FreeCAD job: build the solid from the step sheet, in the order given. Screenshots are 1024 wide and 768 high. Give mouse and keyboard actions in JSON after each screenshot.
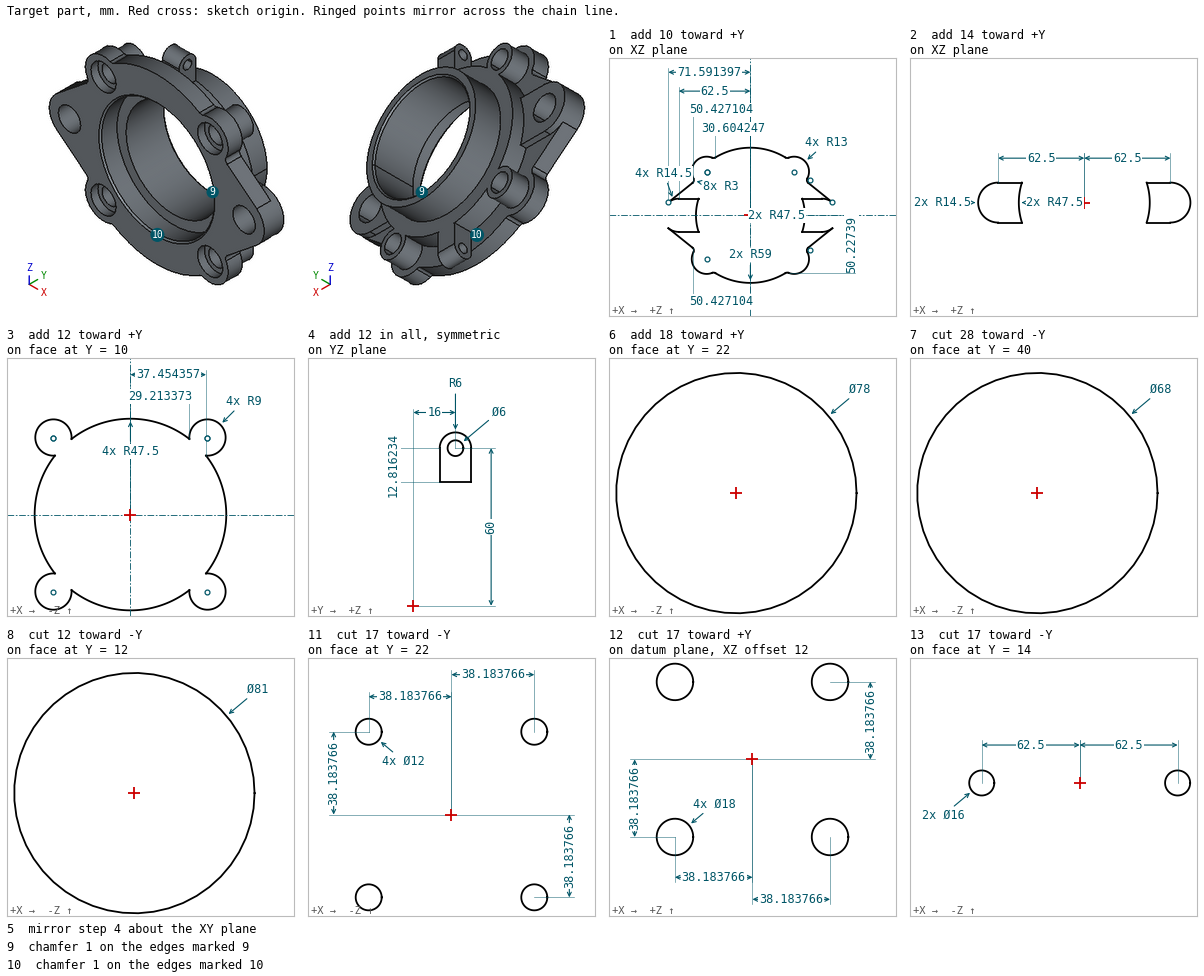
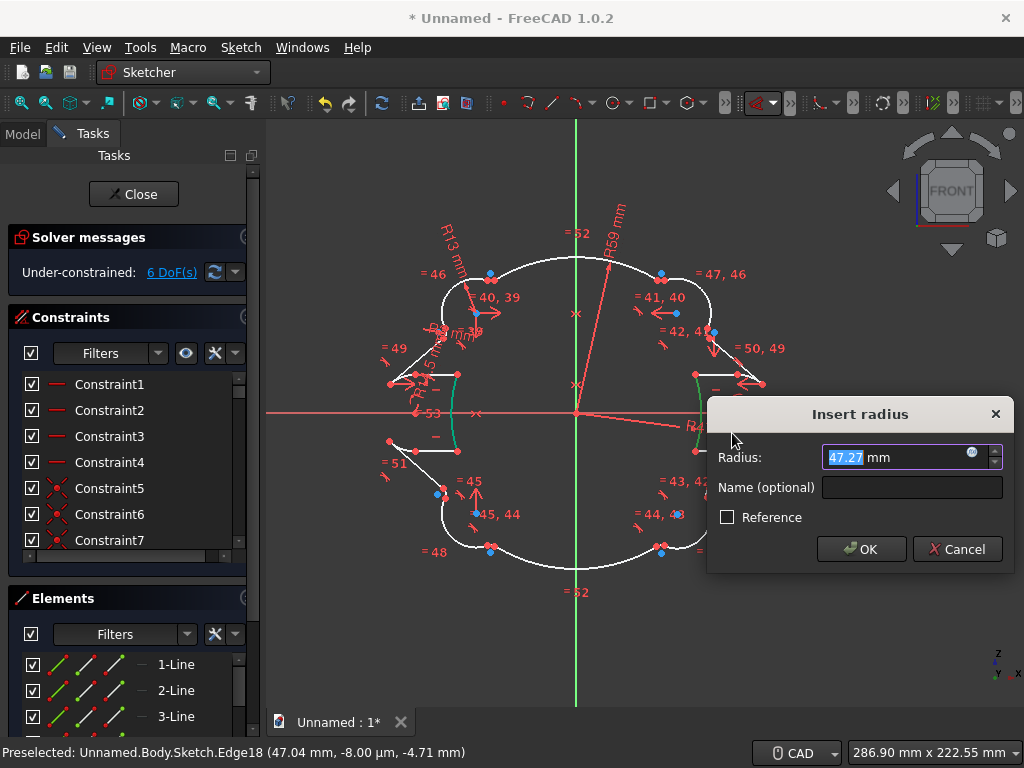
{"action": "type", "text": "47.5"}
{"action": "key", "text": "Return"}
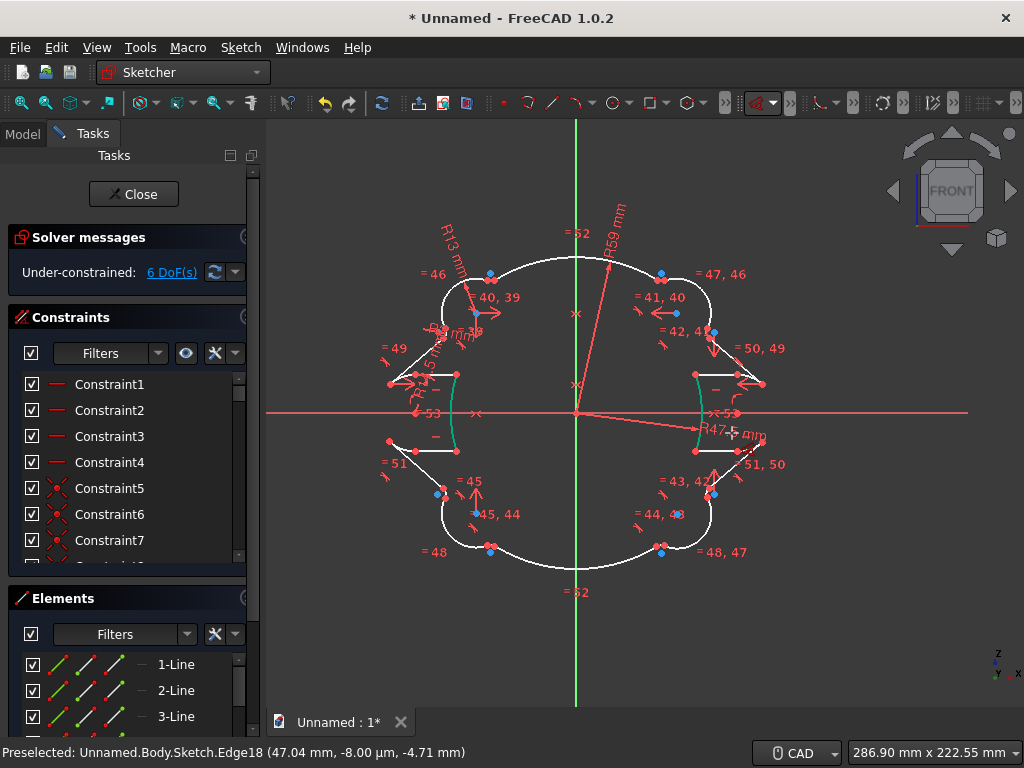
{"action": "left_click", "coordinate": [415, 375]}
{"action": "left_click", "coordinate": [533, 341]}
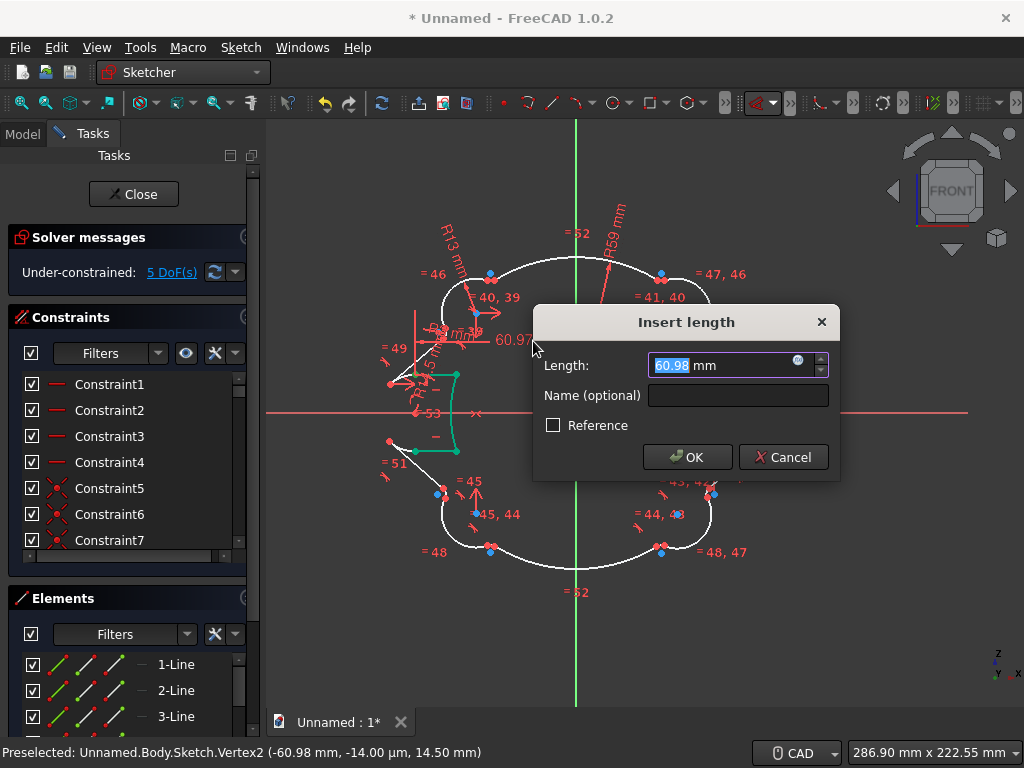
{"action": "type", "text": "62.5"}
{"action": "key", "text": "Return"}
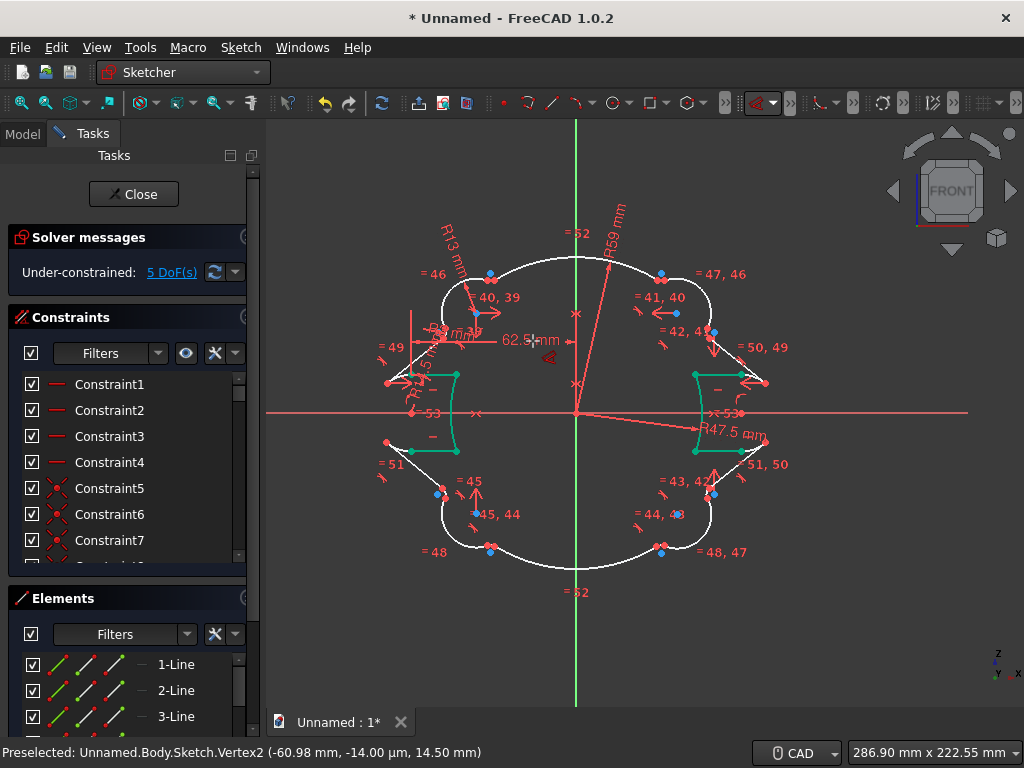
{"action": "scroll", "coordinate": [664, 546], "scroll_direction": "up", "scroll_amount": 3}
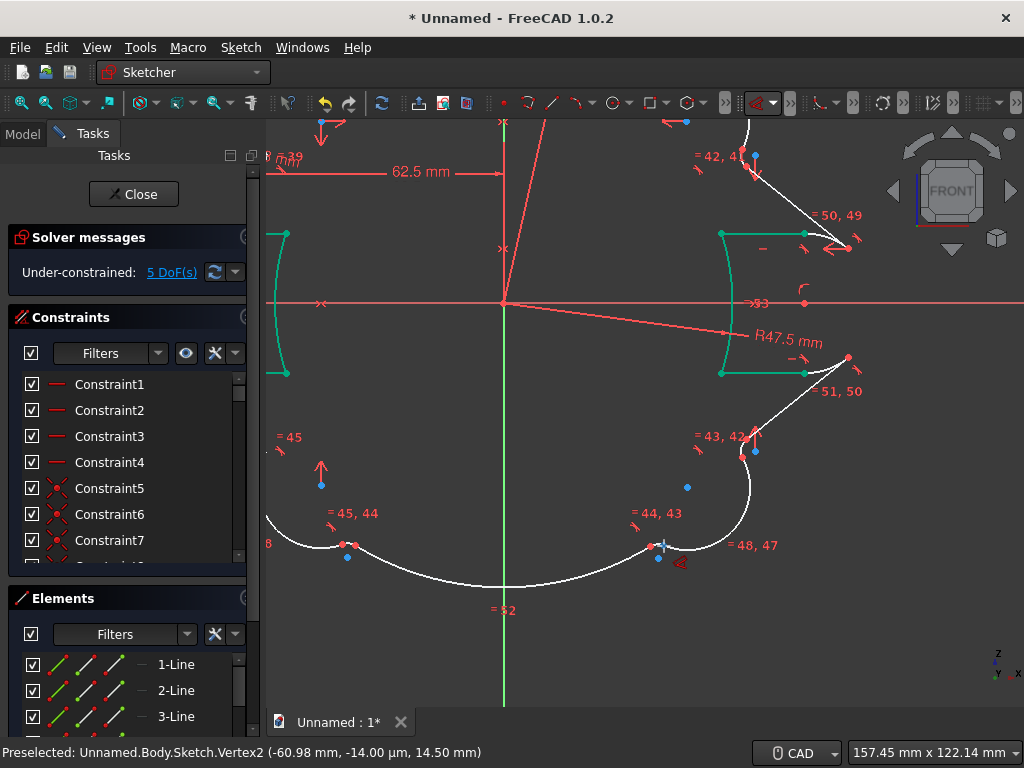
{"action": "left_click", "coordinate": [664, 545]}
{"action": "left_click", "coordinate": [698, 424]}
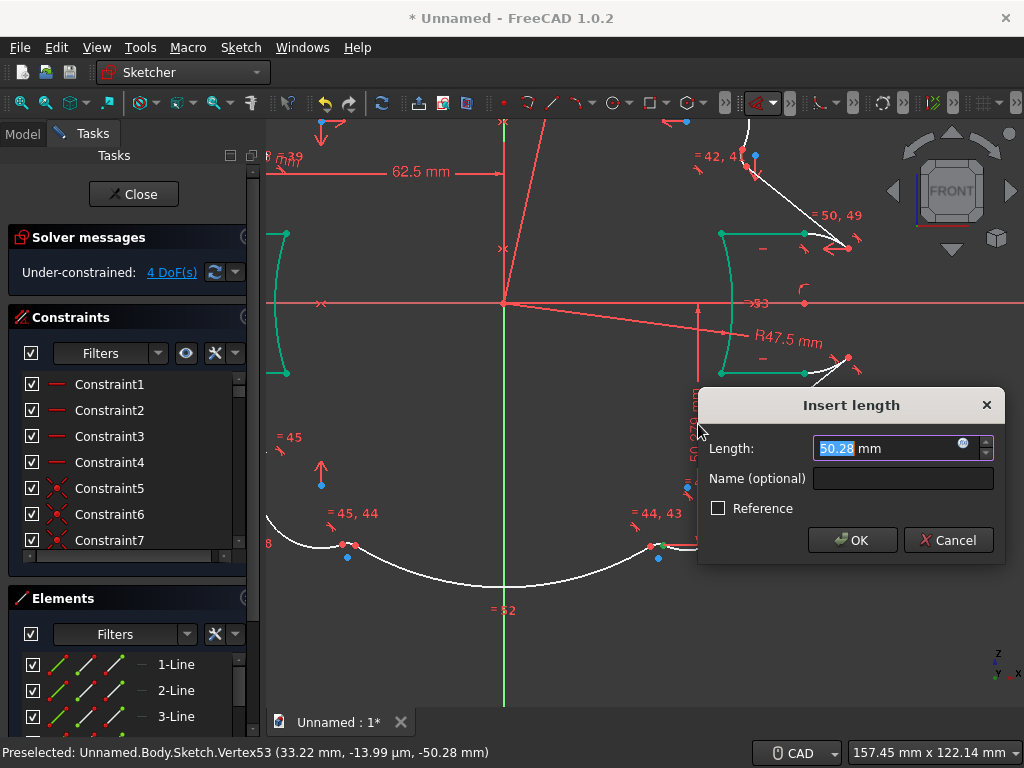
{"action": "type", "text": "50.22739"}
{"action": "key", "text": "Return"}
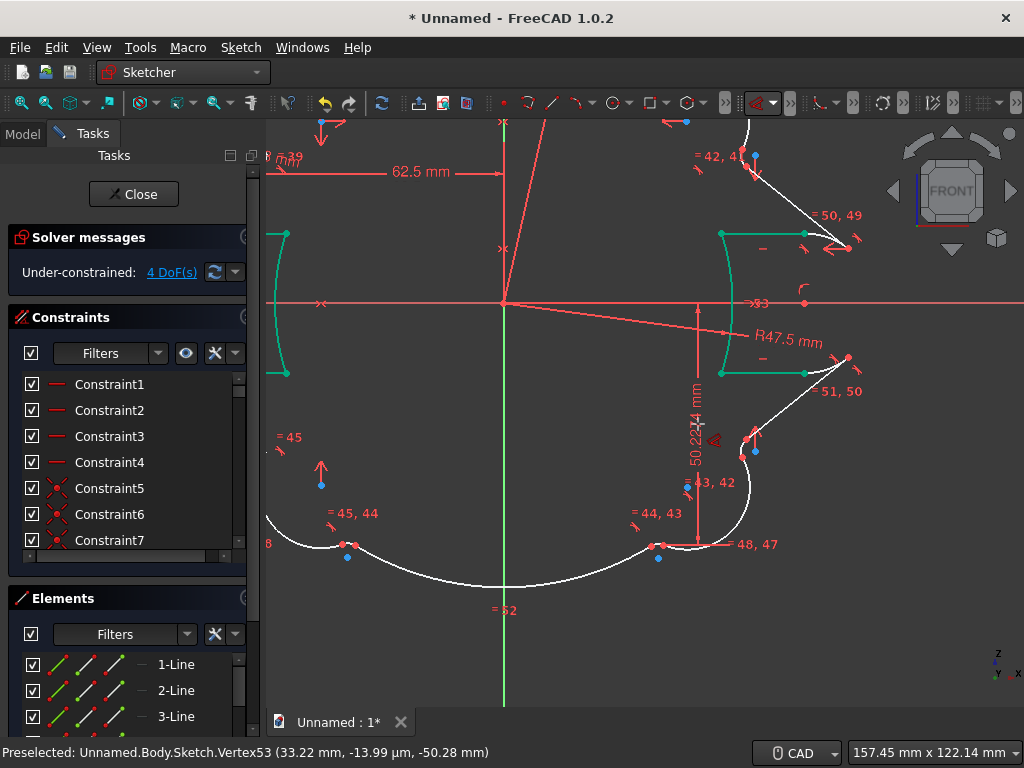
{"action": "scroll", "coordinate": [665, 546], "scroll_direction": "down", "scroll_amount": 3}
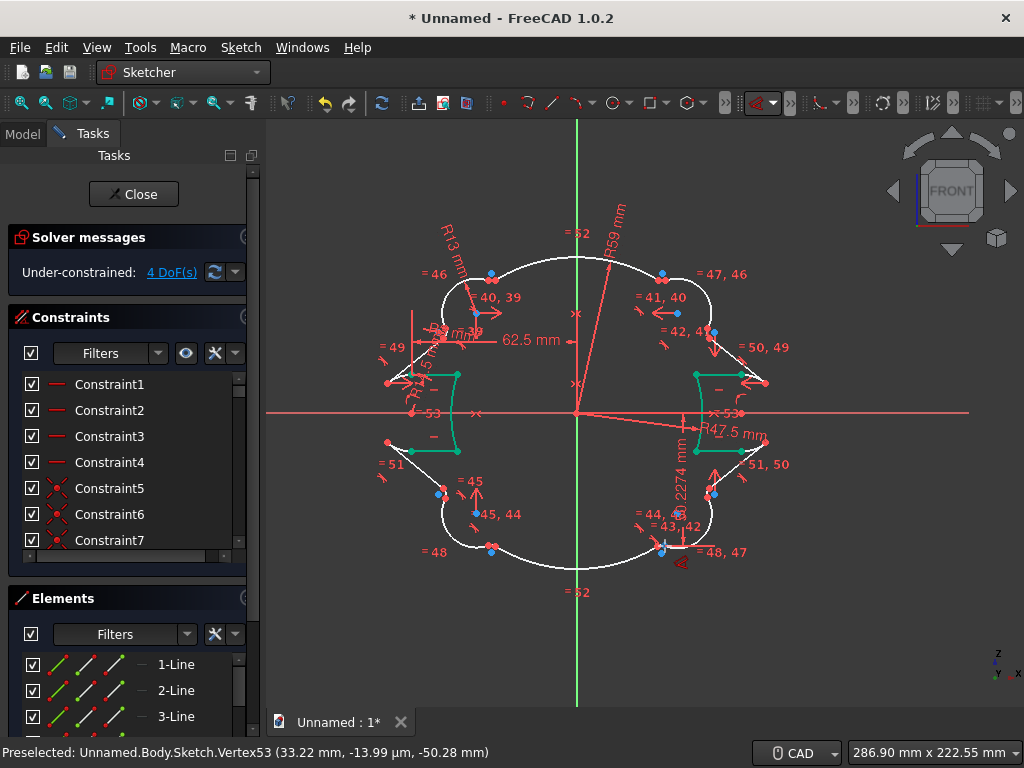
{"action": "left_click", "coordinate": [388, 383]}
{"action": "left_click", "coordinate": [482, 447]}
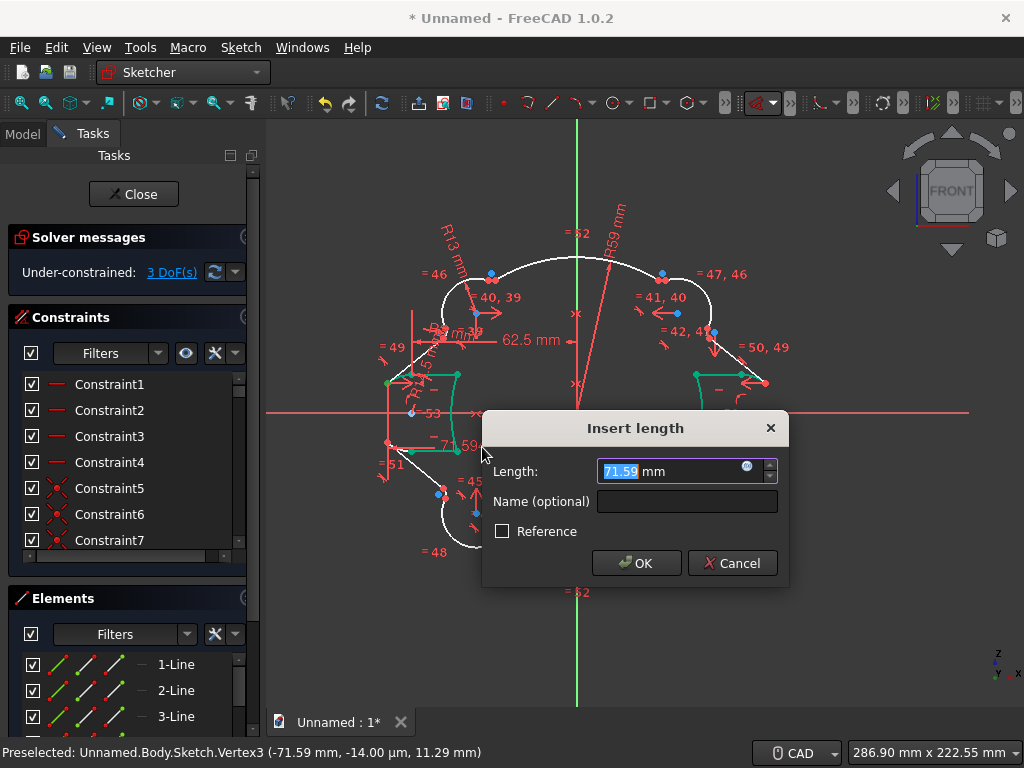
{"action": "type", "text": "71.591397"}
{"action": "key", "text": "Return"}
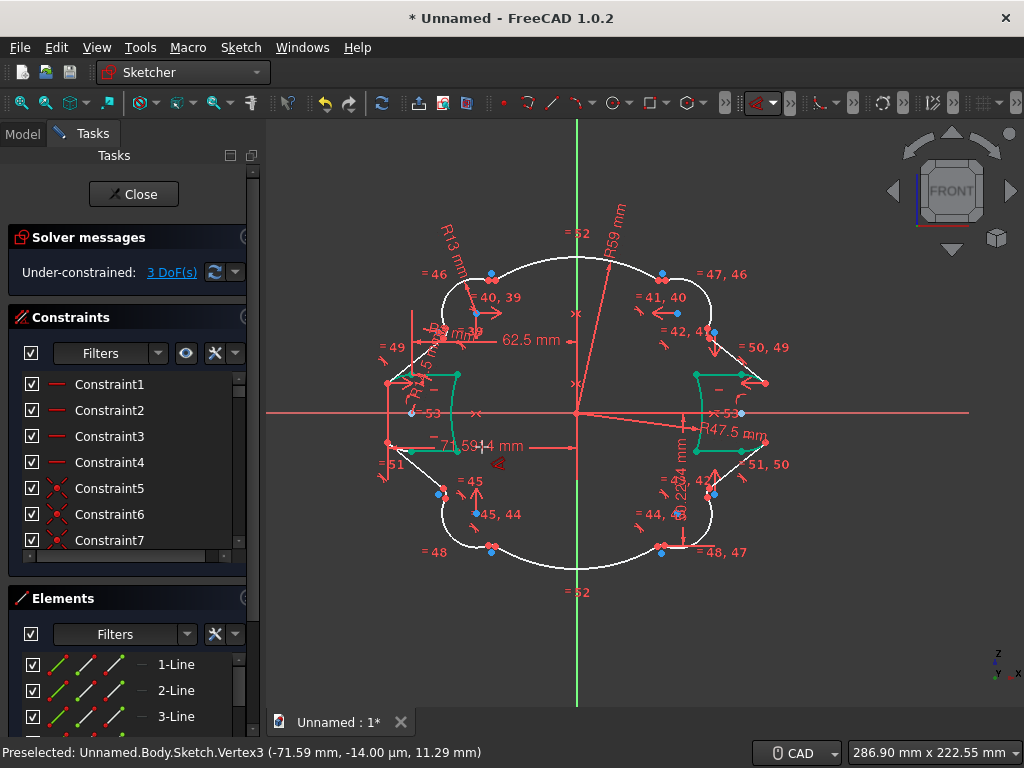
{"action": "scroll", "coordinate": [444, 338], "scroll_direction": "up", "scroll_amount": 3}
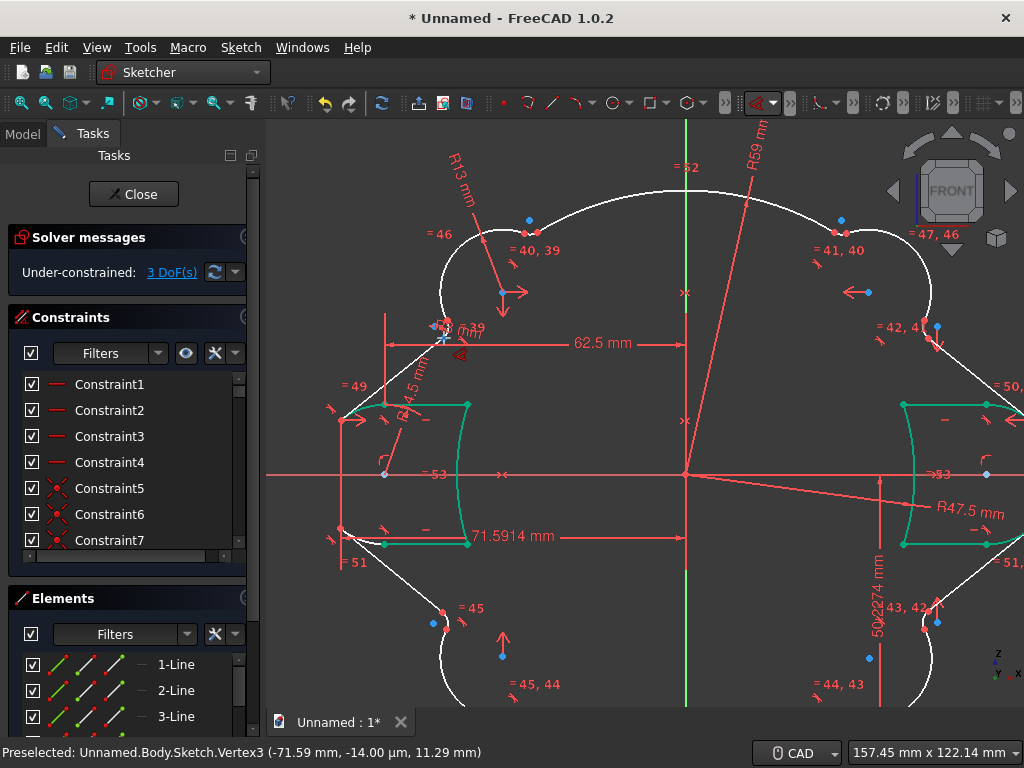
{"action": "left_click", "coordinate": [443, 338]}
{"action": "left_click", "coordinate": [564, 304]}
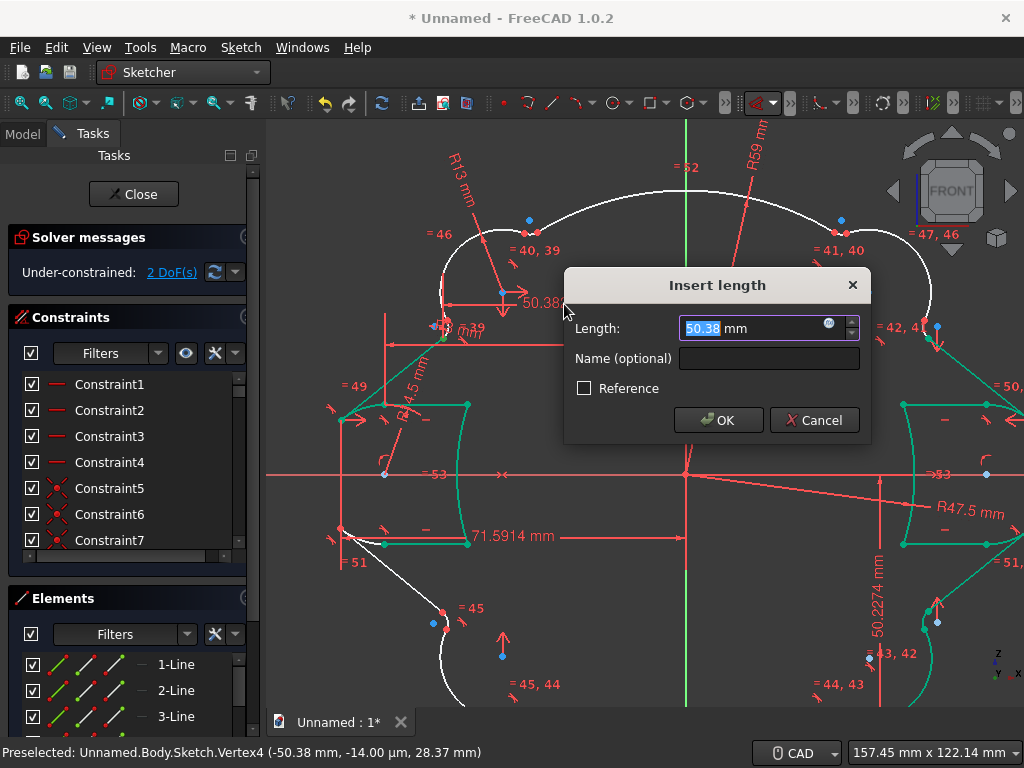
{"action": "type", "text": "50.427104"}
{"action": "key", "text": "Return"}